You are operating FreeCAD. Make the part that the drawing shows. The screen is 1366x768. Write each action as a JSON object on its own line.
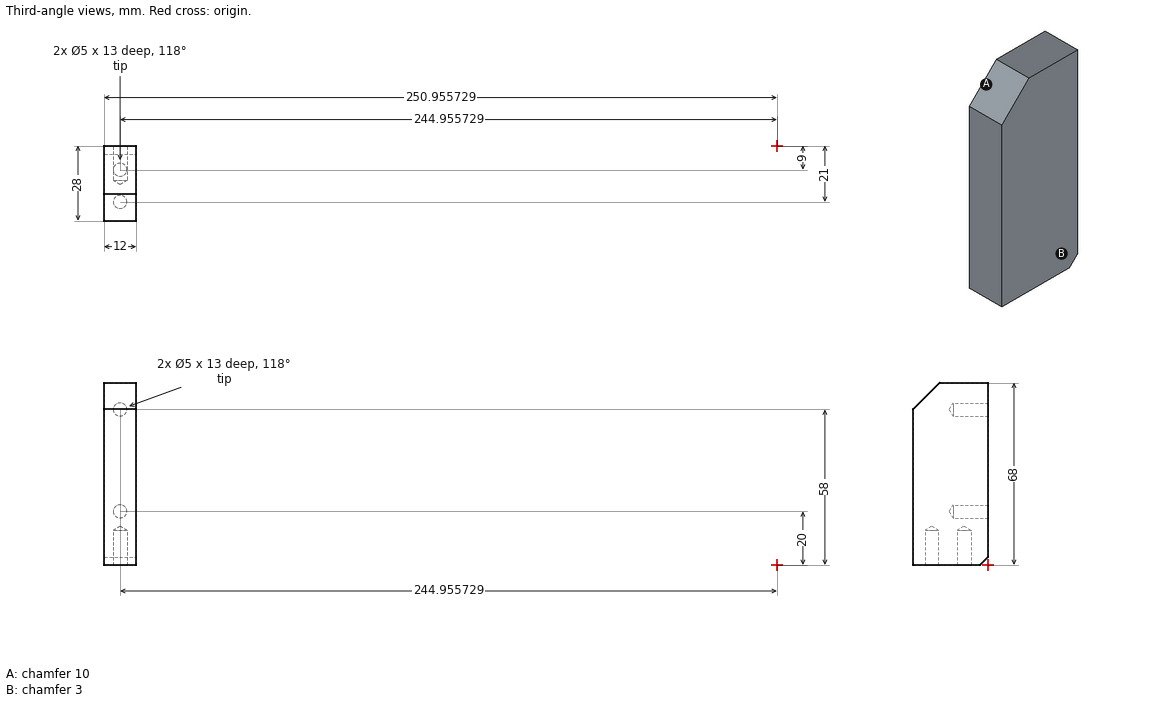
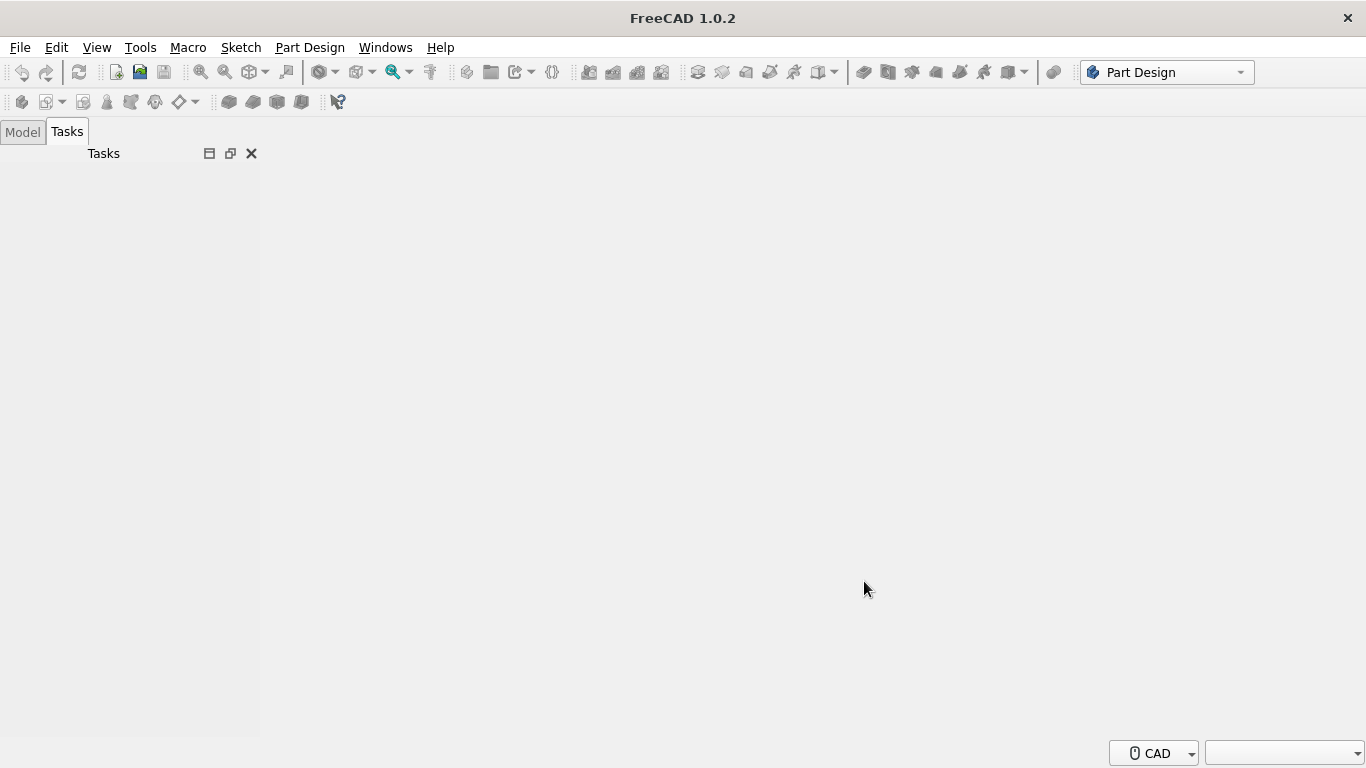
{"action": "key", "text": "ctrl+n"}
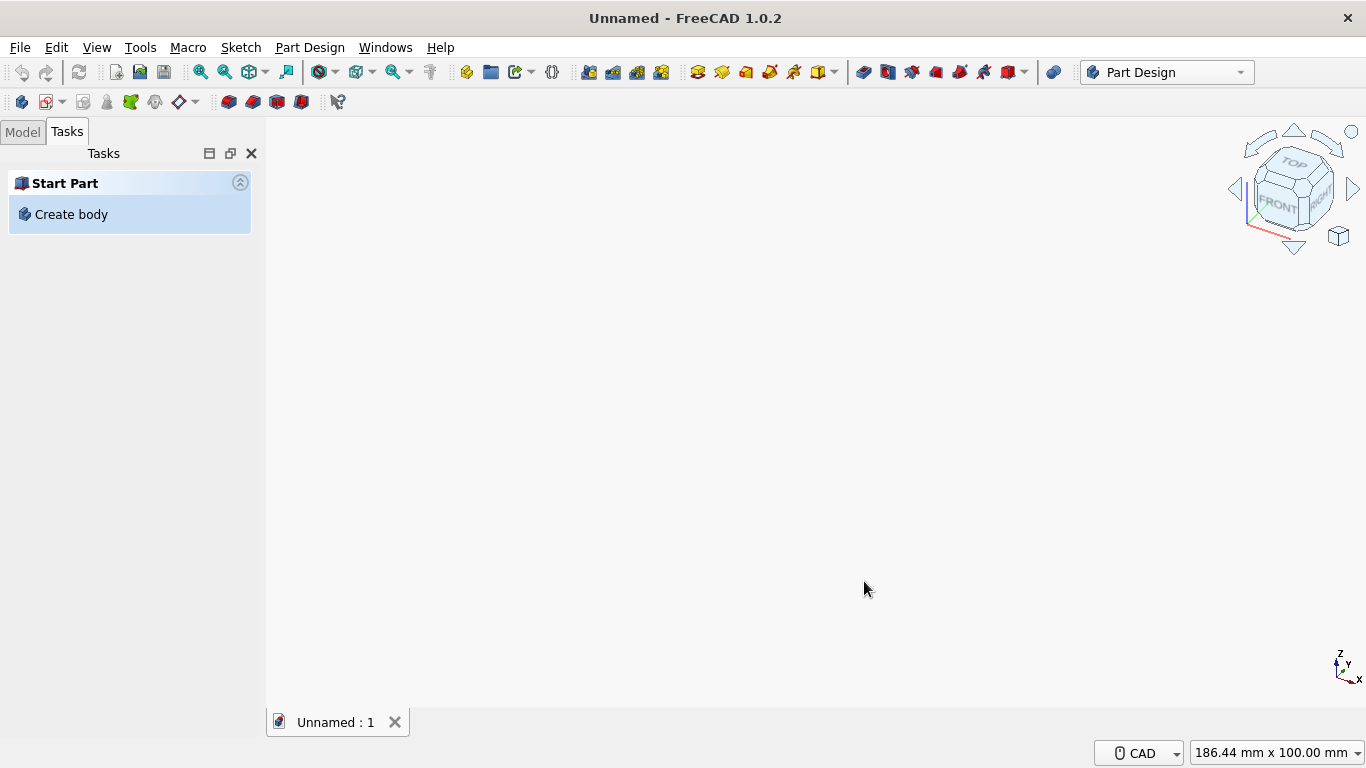
{"action": "left_click", "coordinate": [46, 102]}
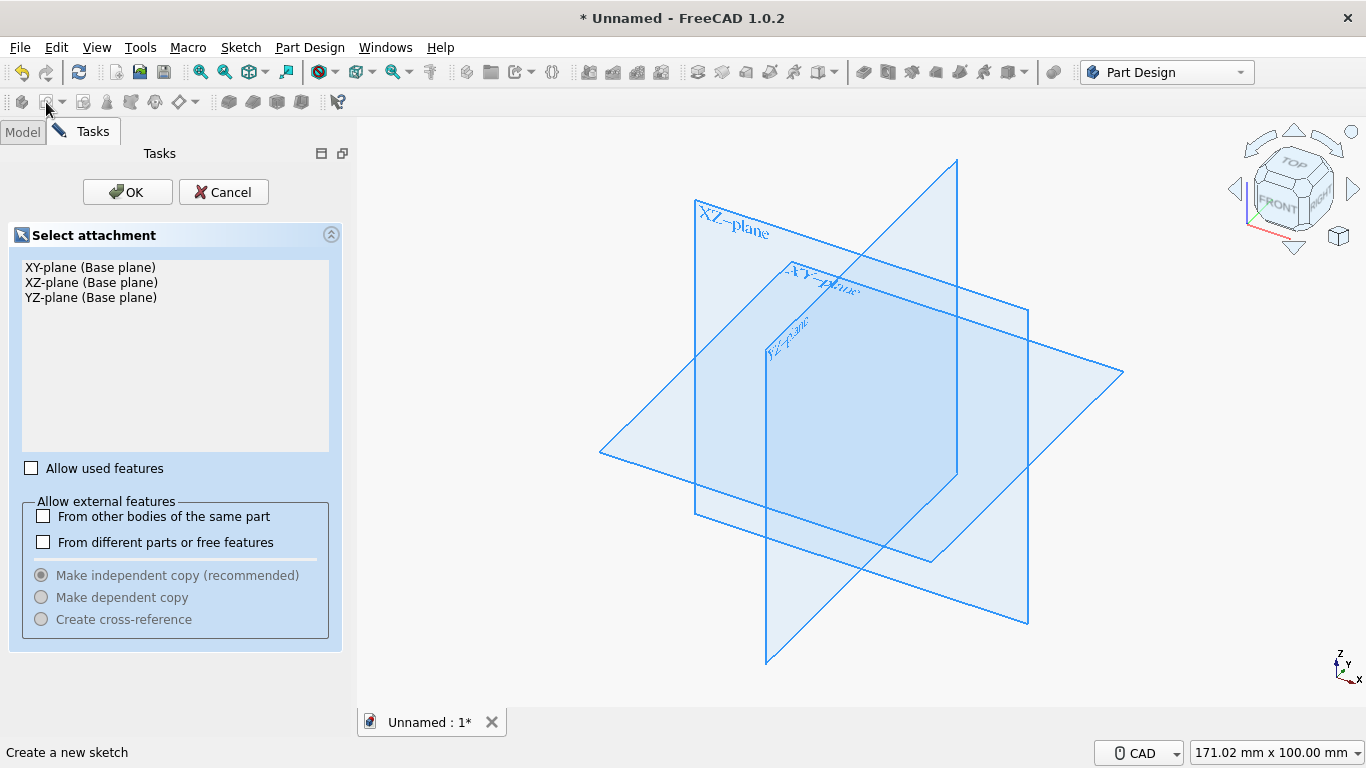
{"action": "left_click", "coordinate": [82, 268]}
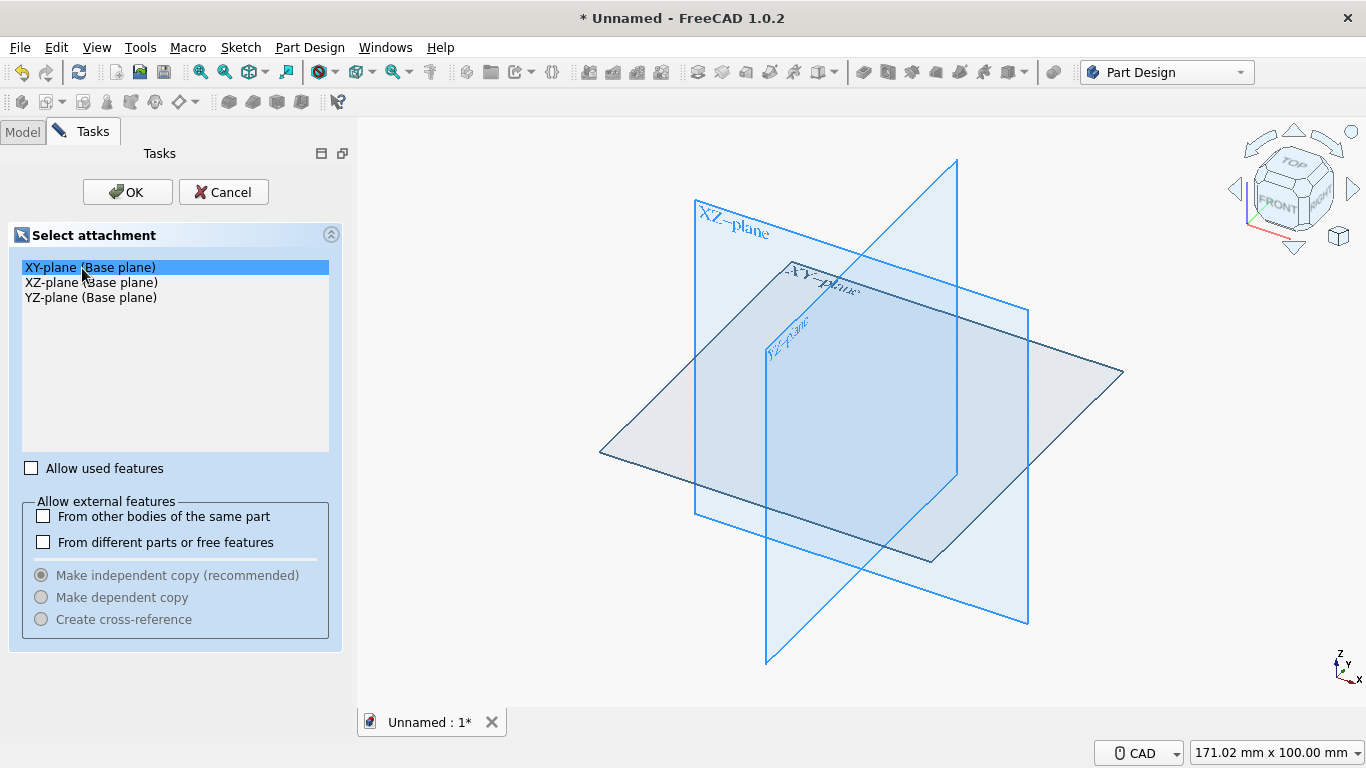
{"action": "left_click", "coordinate": [128, 192]}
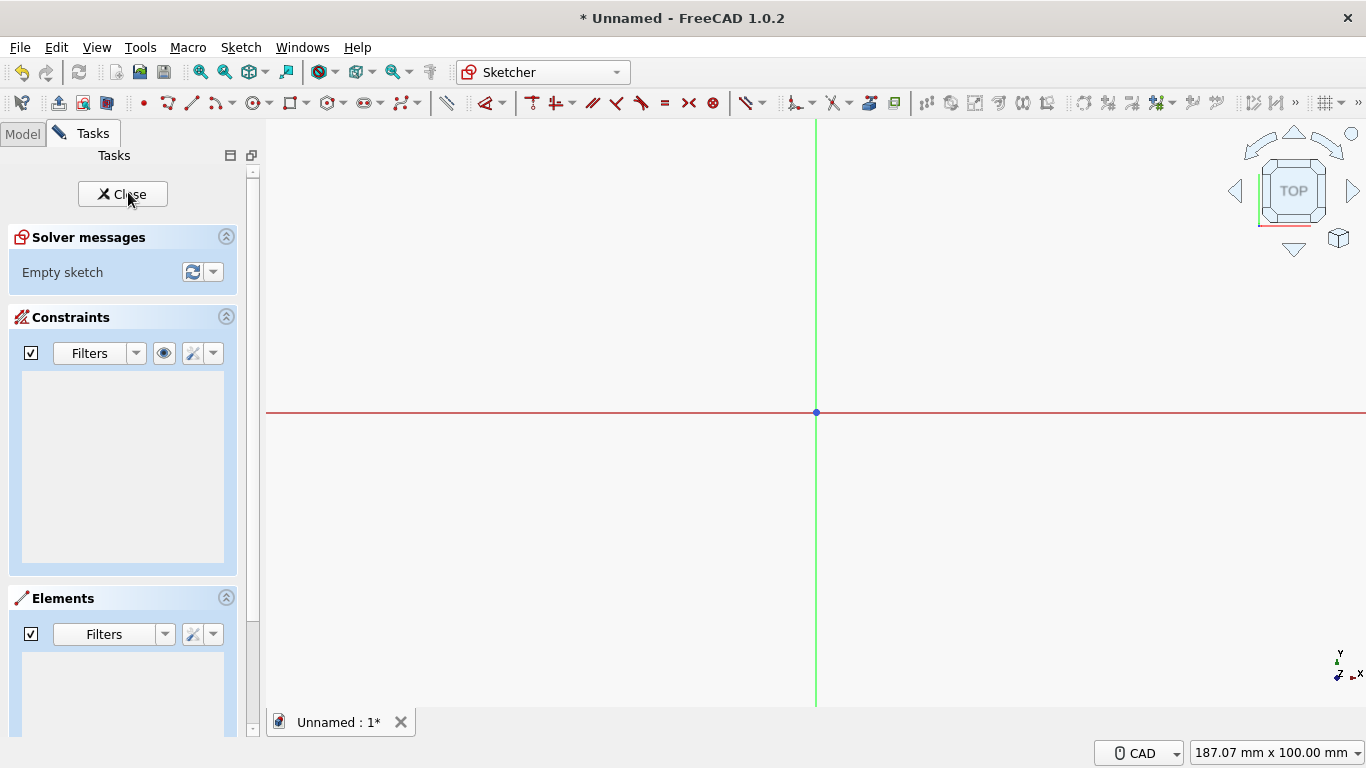
{"action": "scroll", "coordinate": [748, 413], "scroll_direction": "down", "scroll_amount": 5}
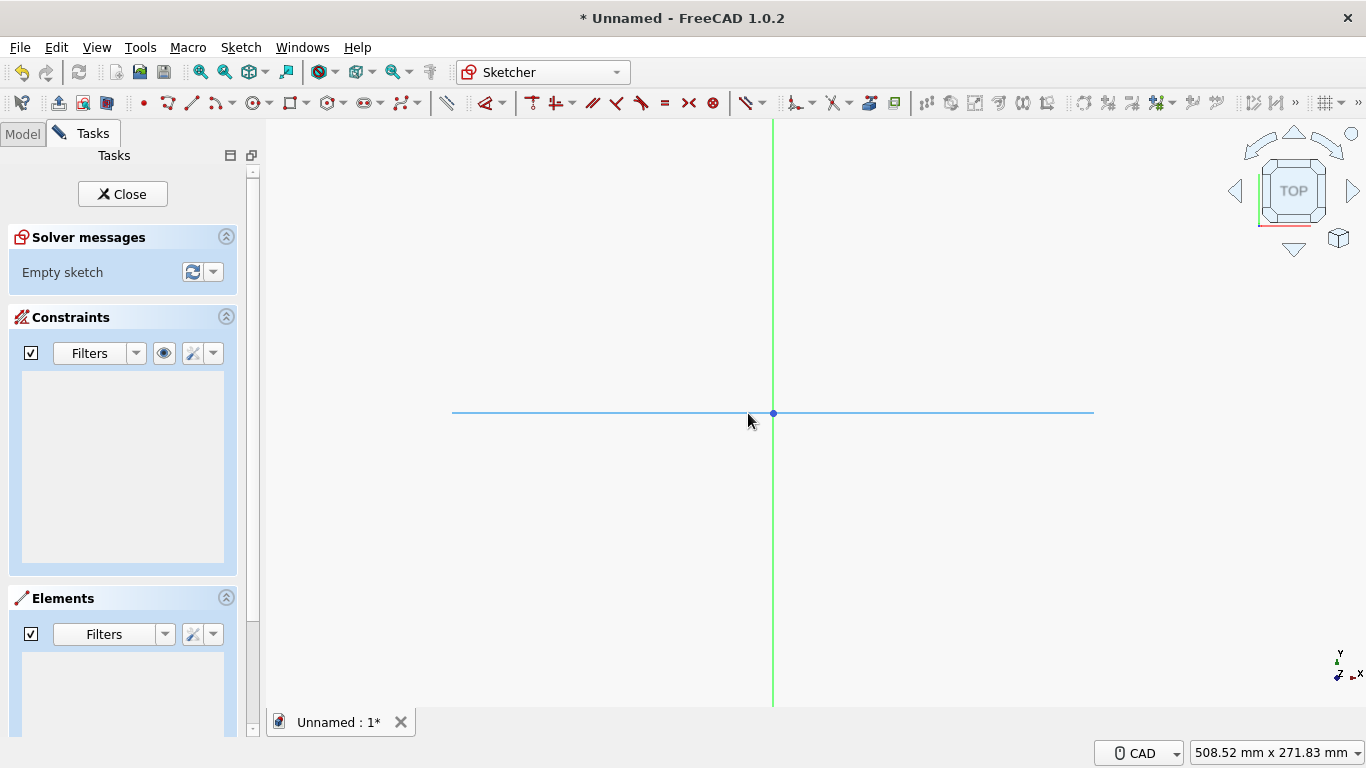
{"action": "scroll", "coordinate": [748, 413], "scroll_direction": "down", "scroll_amount": 5}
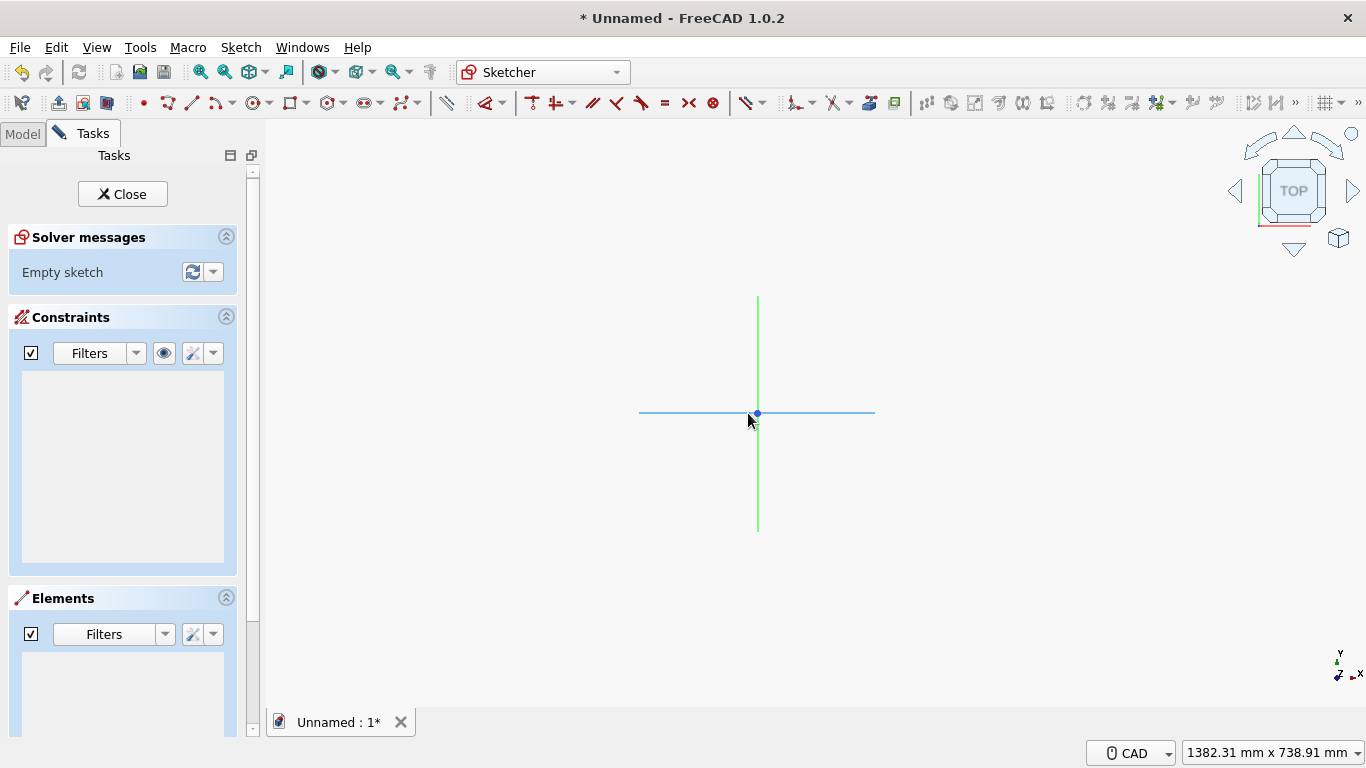
{"action": "scroll", "coordinate": [551, 425], "scroll_direction": "up", "scroll_amount": 14}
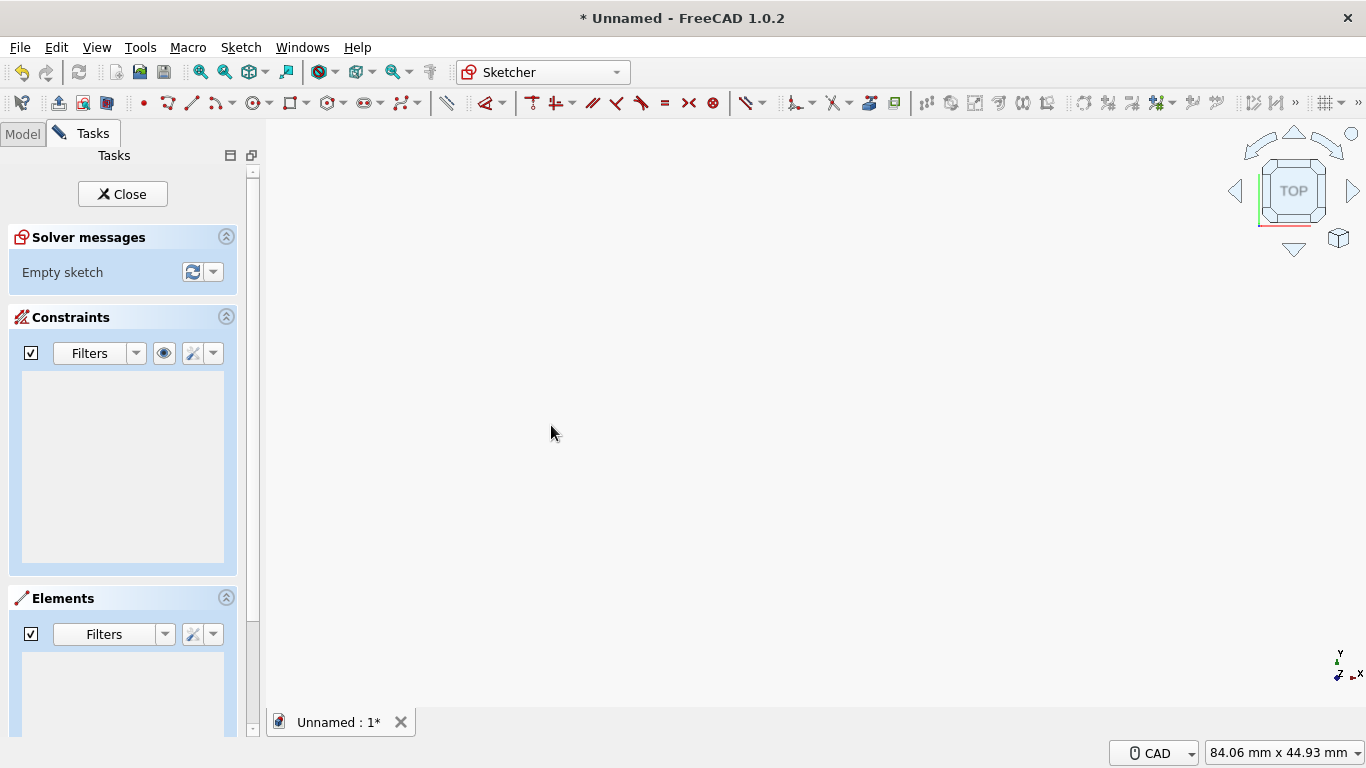
{"action": "left_click", "coordinate": [290, 104]}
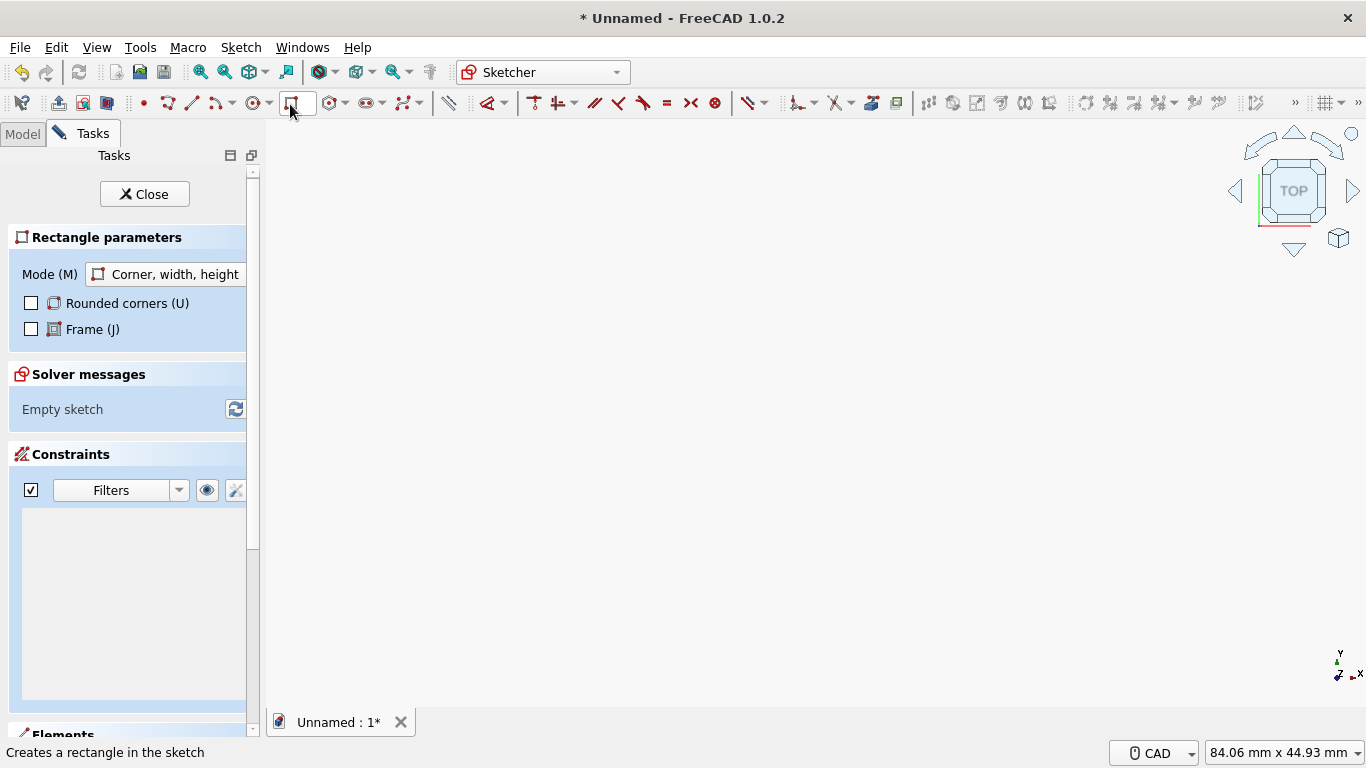
{"action": "left_click", "coordinate": [660, 227]}
{"action": "mouse_move", "coordinate": [817, 593]}